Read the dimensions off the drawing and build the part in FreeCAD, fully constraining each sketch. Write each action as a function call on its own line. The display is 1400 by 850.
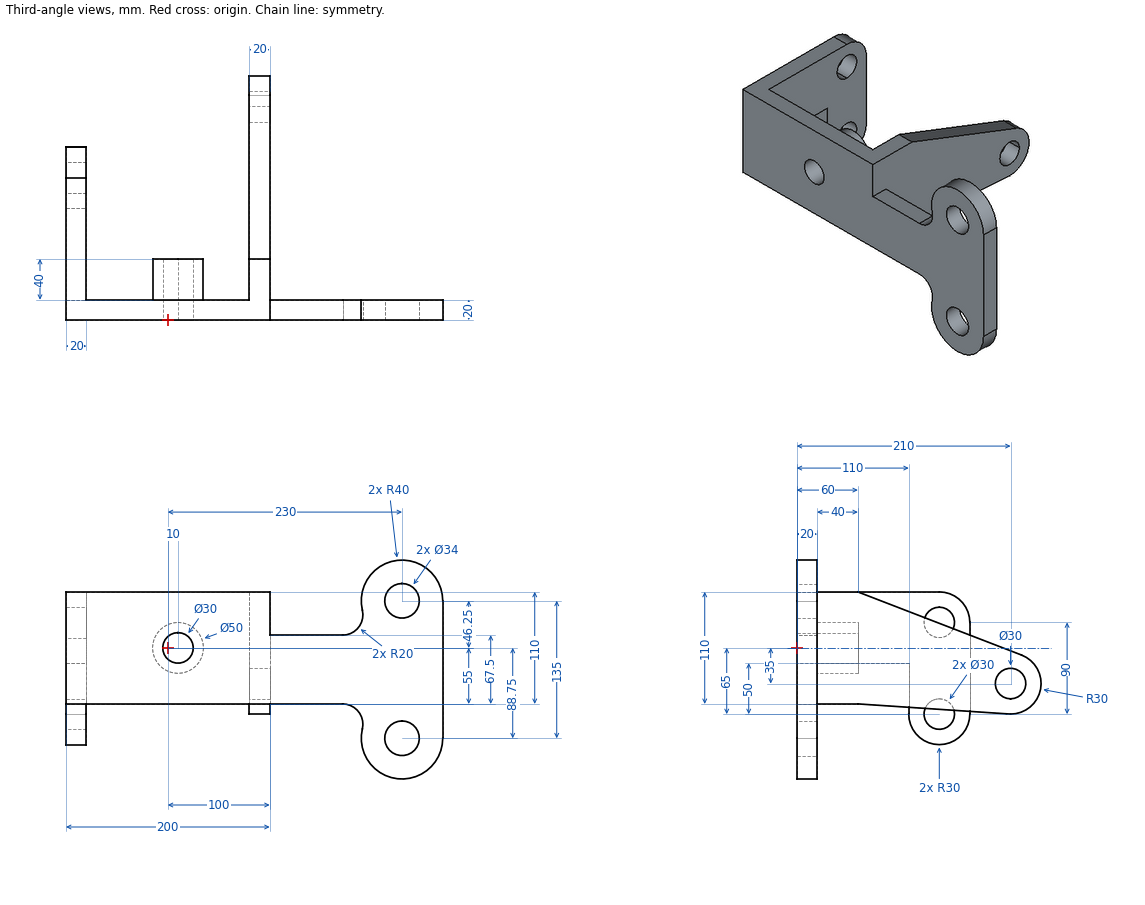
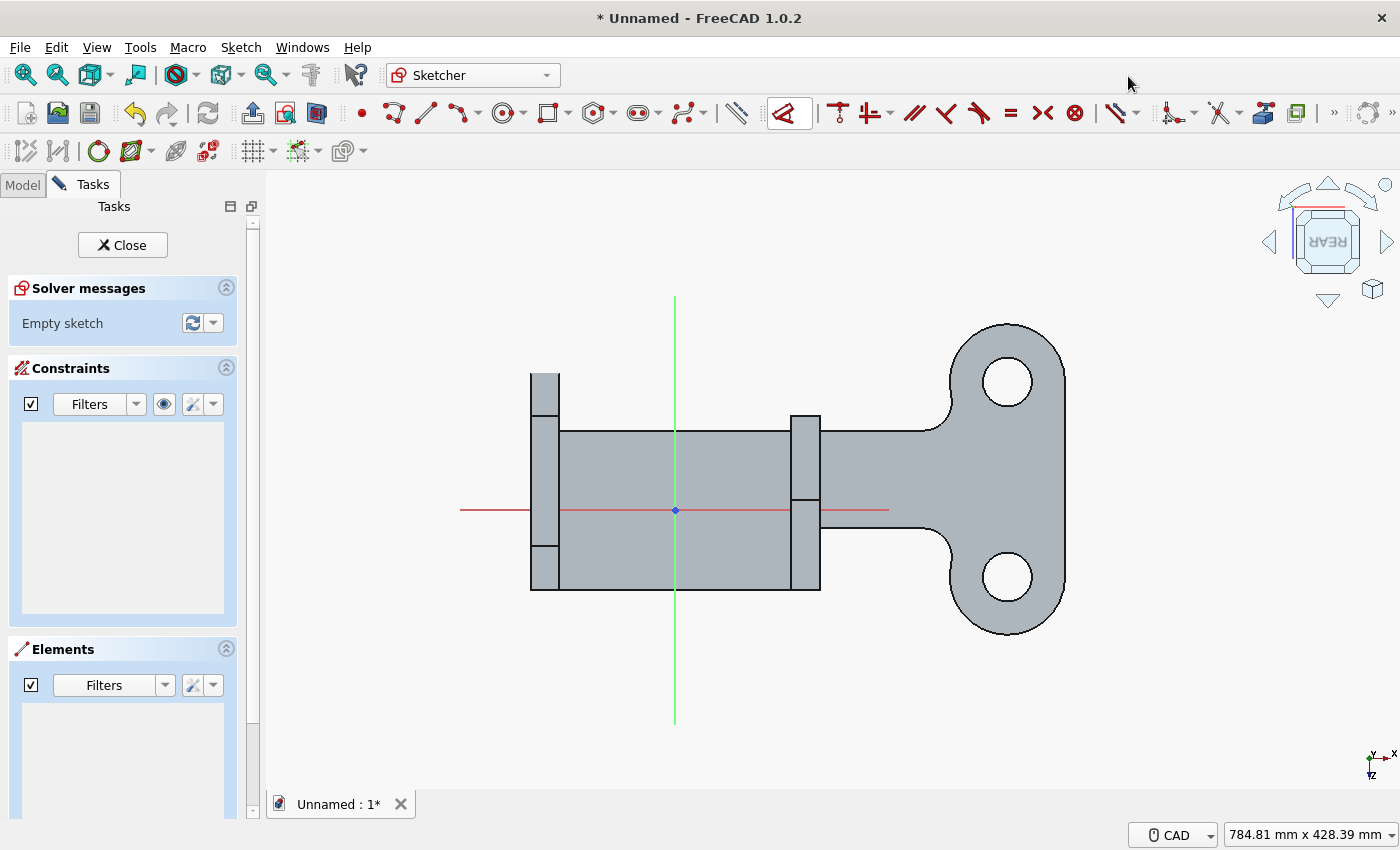
scroll(675, 516, up, 9)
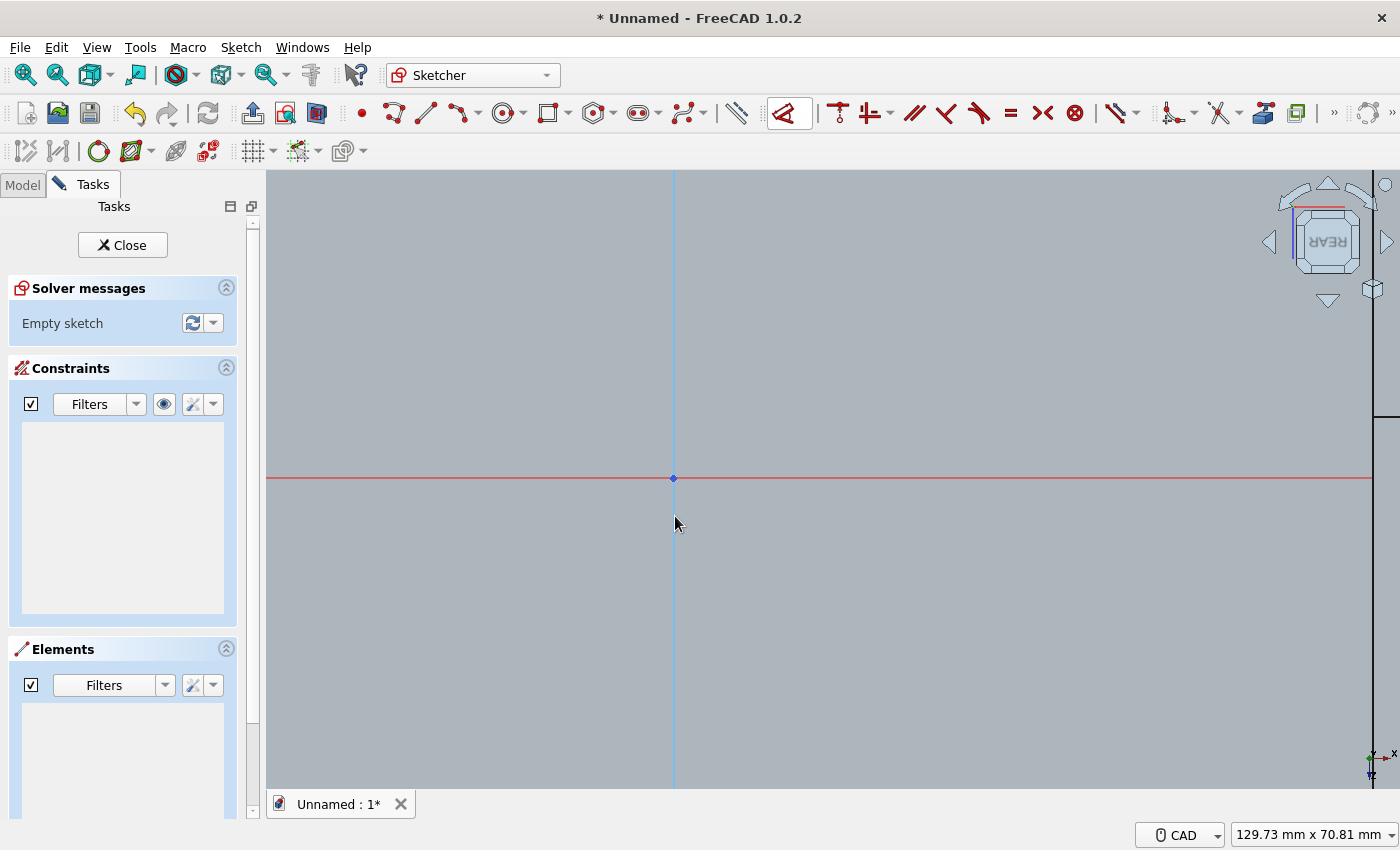
click(504, 114)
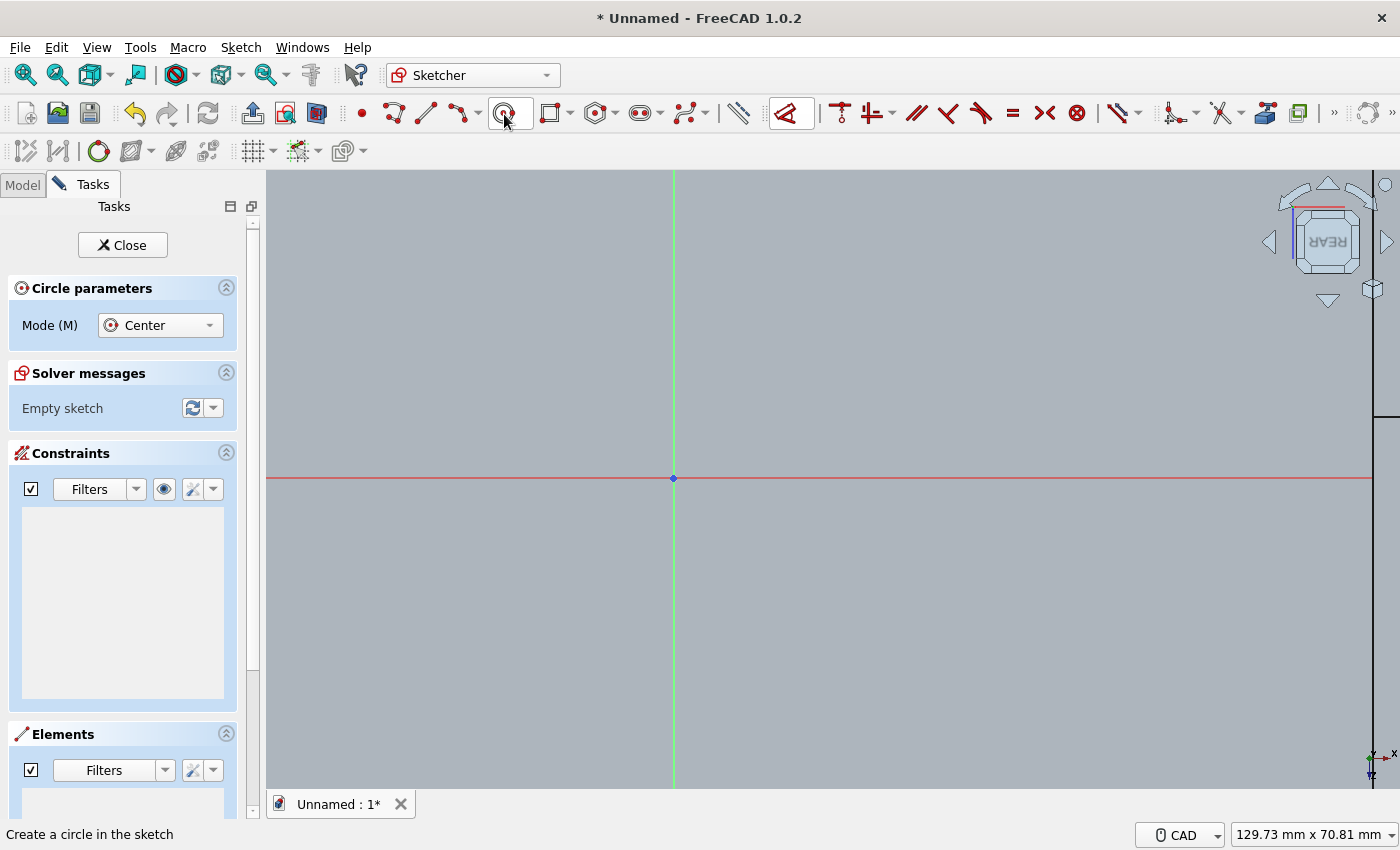
click(761, 478)
click(916, 324)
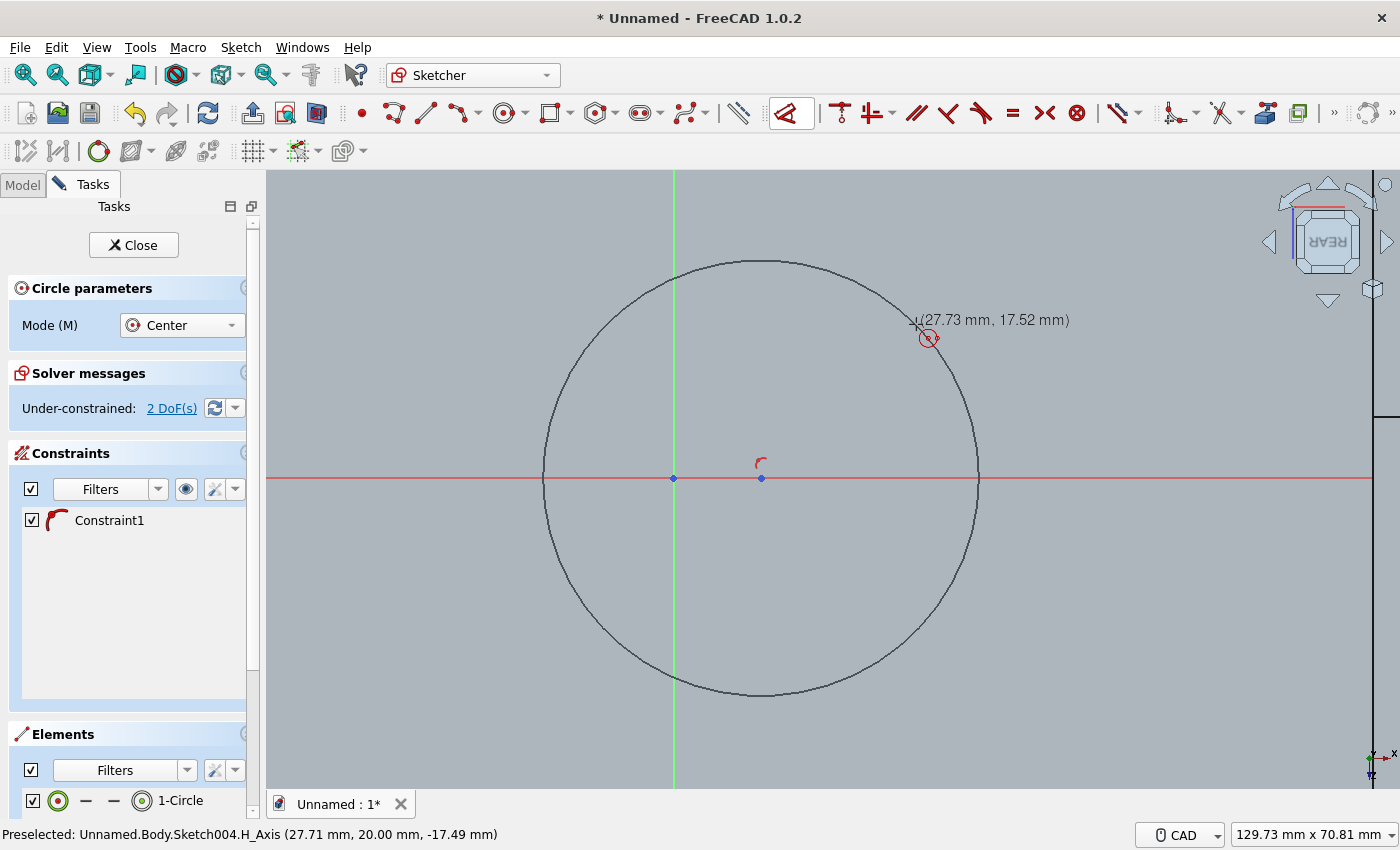
click(761, 478)
click(854, 385)
key(Escape)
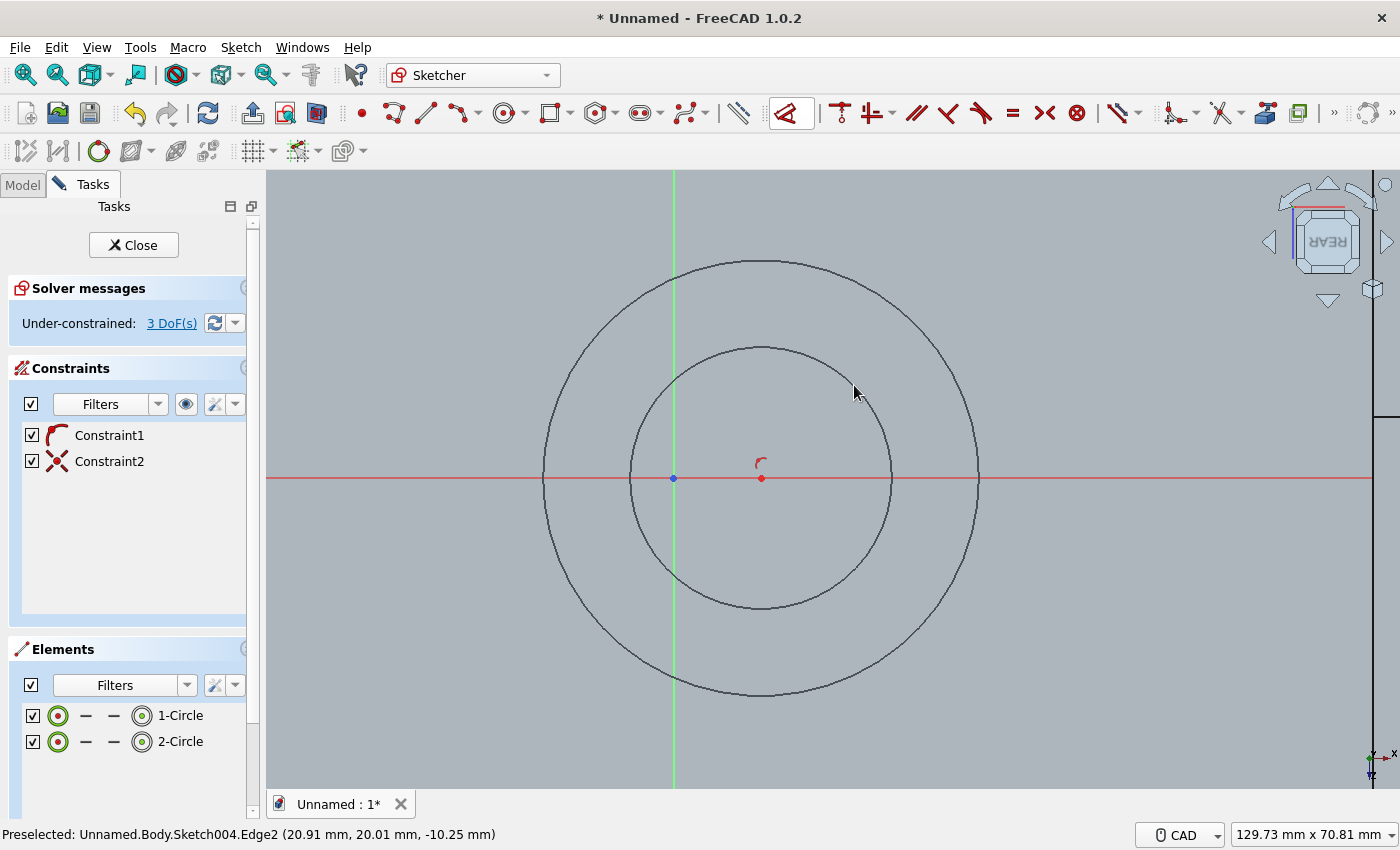
click(915, 324)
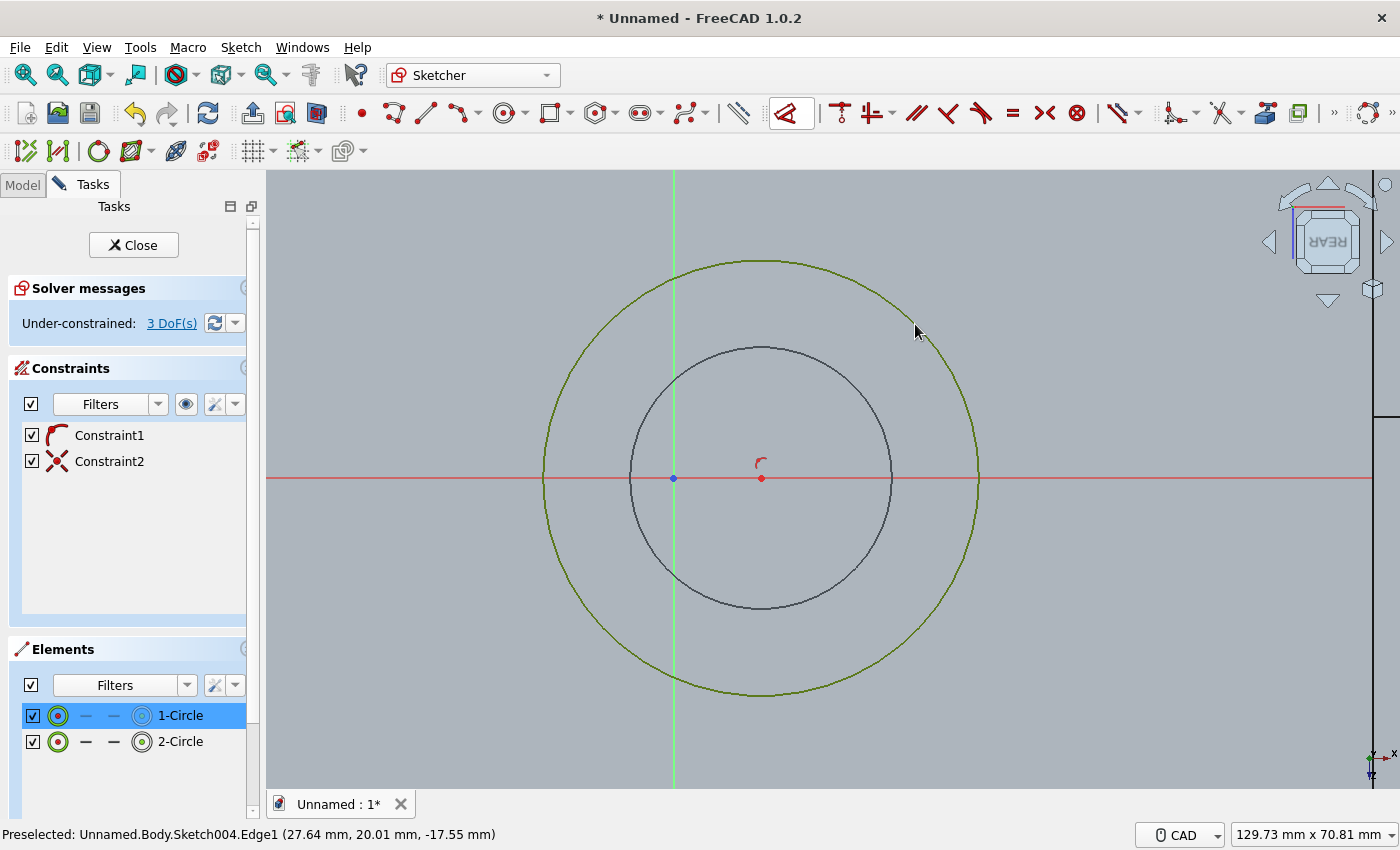
key(k)
key(o)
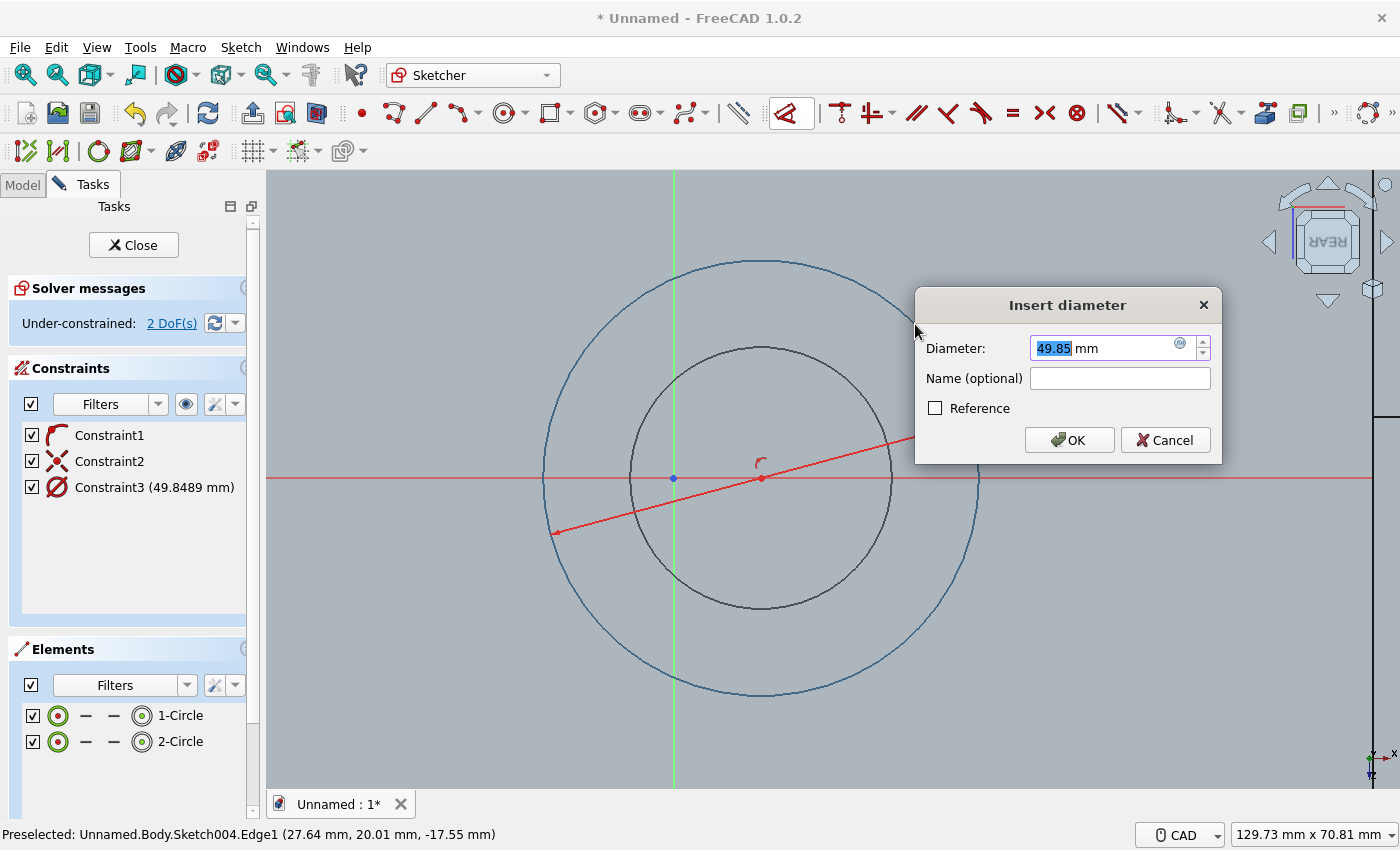
text(50)
key(Return)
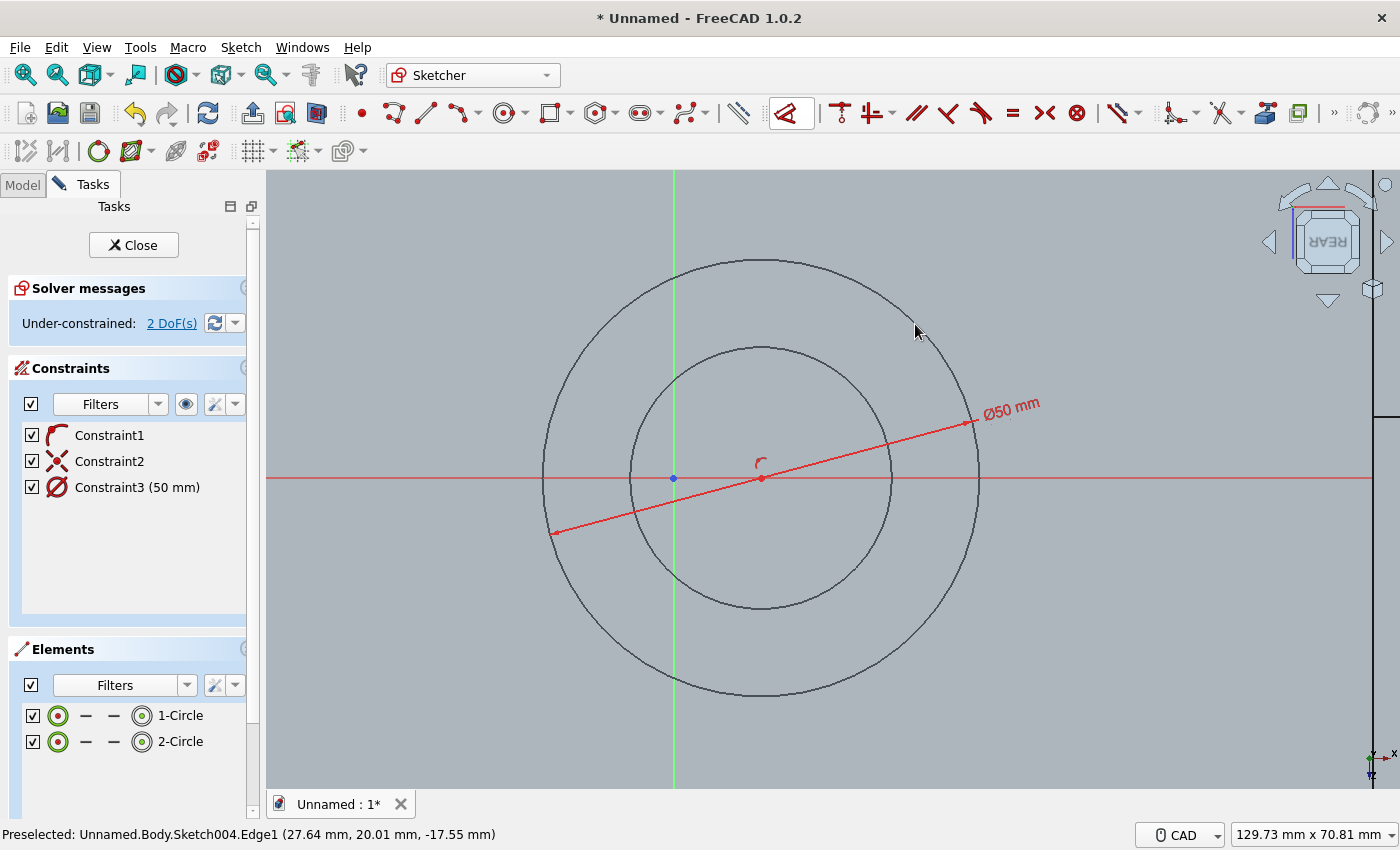
click(853, 385)